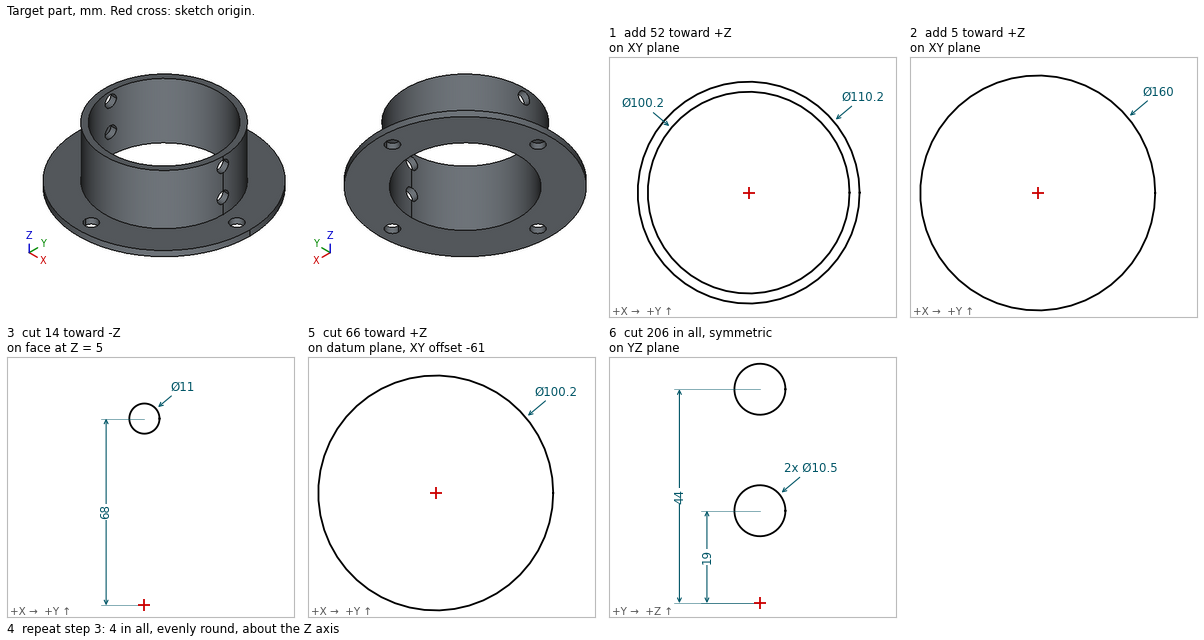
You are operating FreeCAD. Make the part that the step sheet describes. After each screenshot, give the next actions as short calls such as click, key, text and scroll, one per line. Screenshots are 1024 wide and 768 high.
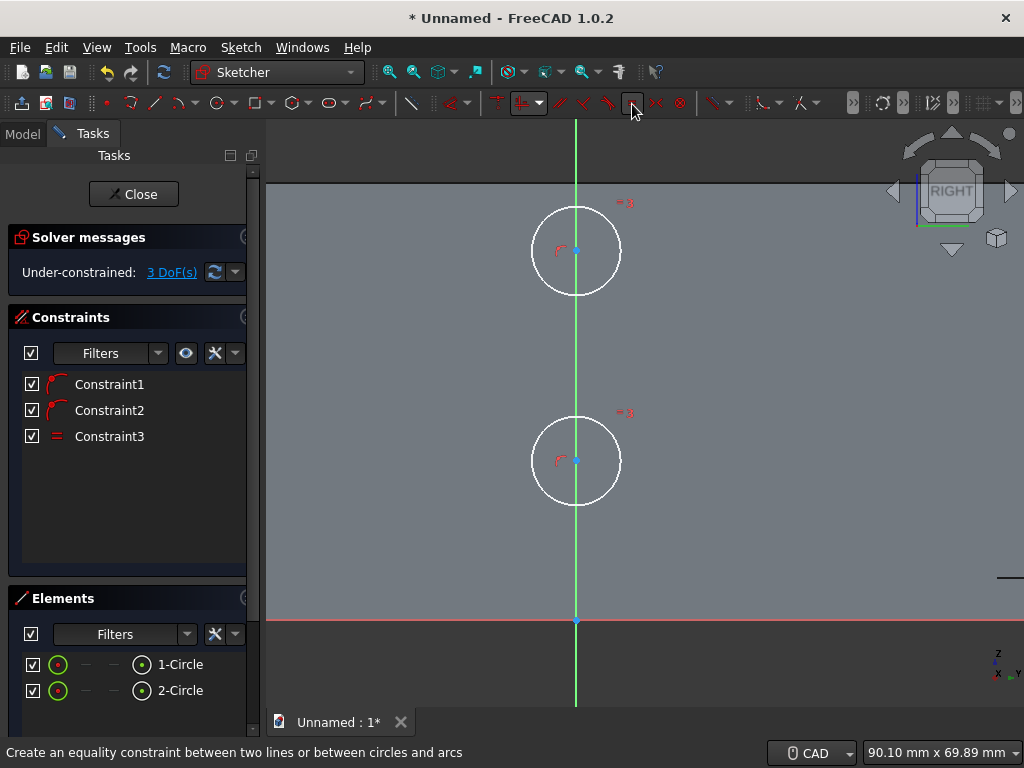
click(450, 104)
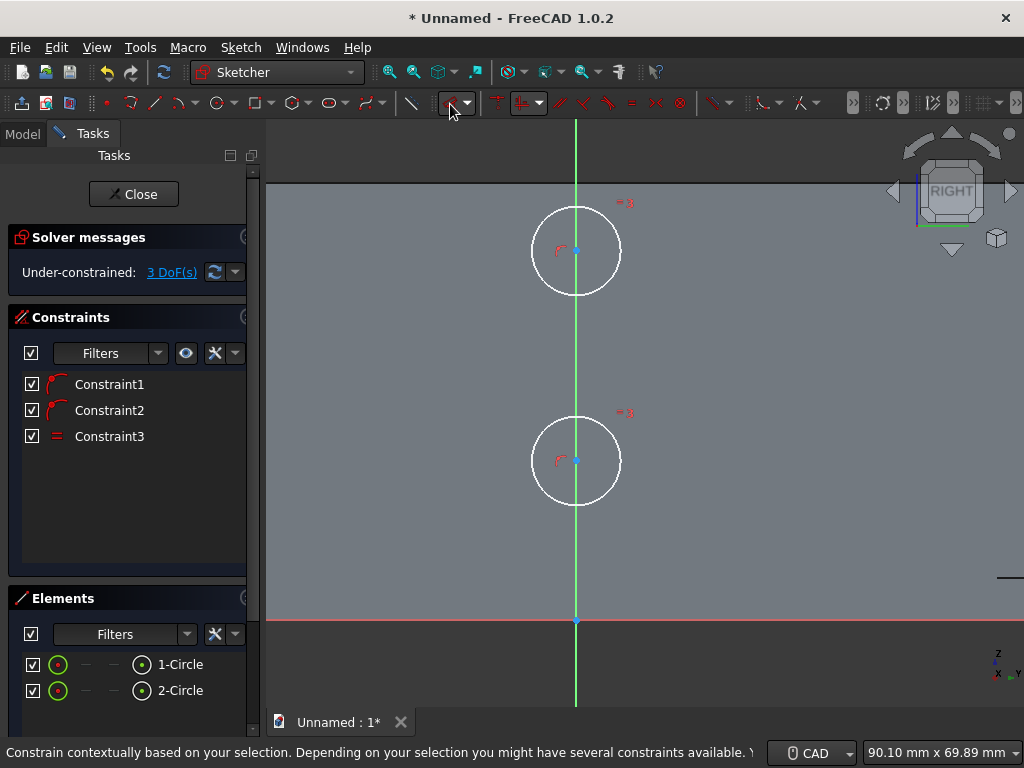
click(608, 430)
click(631, 408)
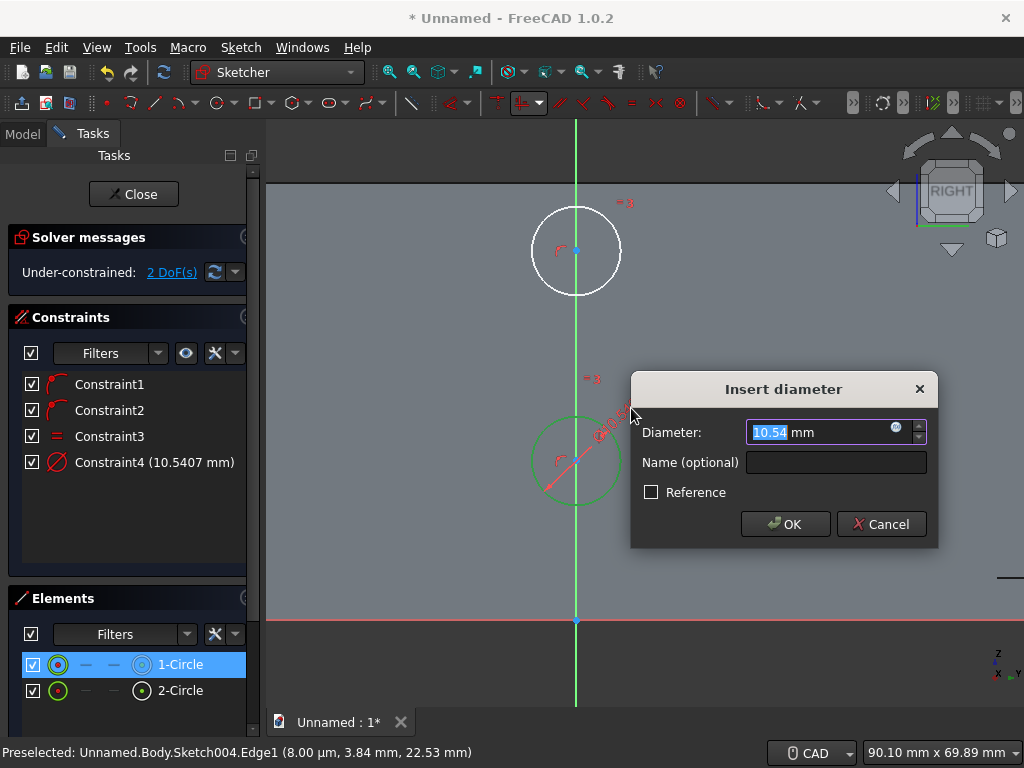
text(10.5)
key(Return)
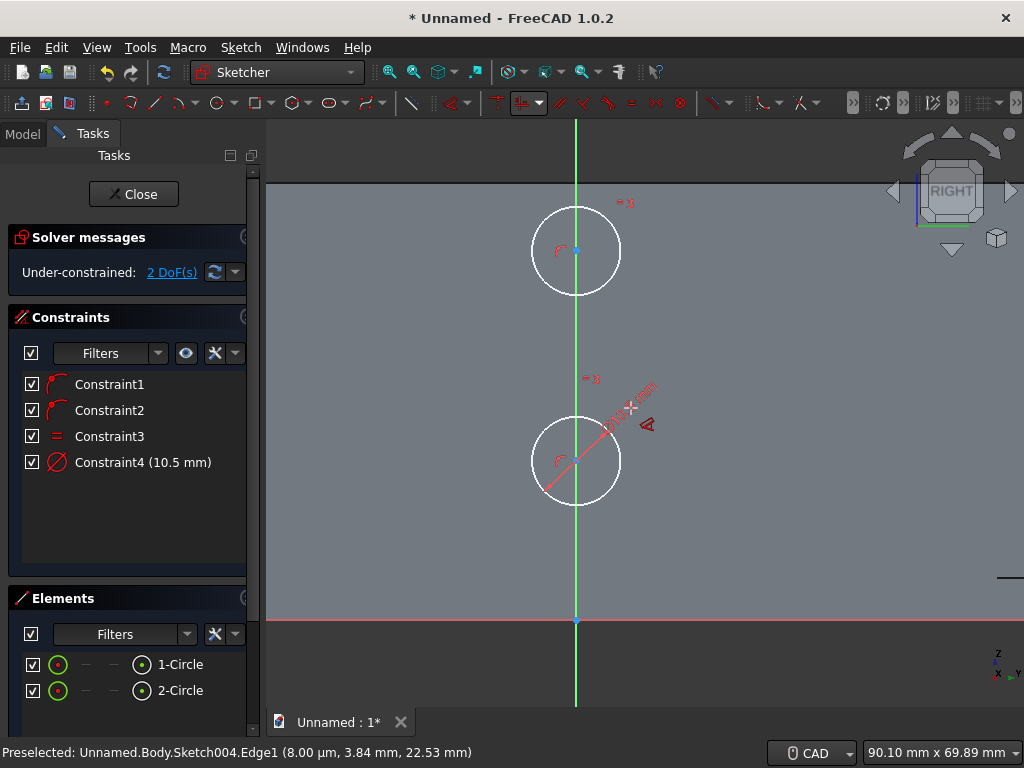
click(576, 461)
click(610, 541)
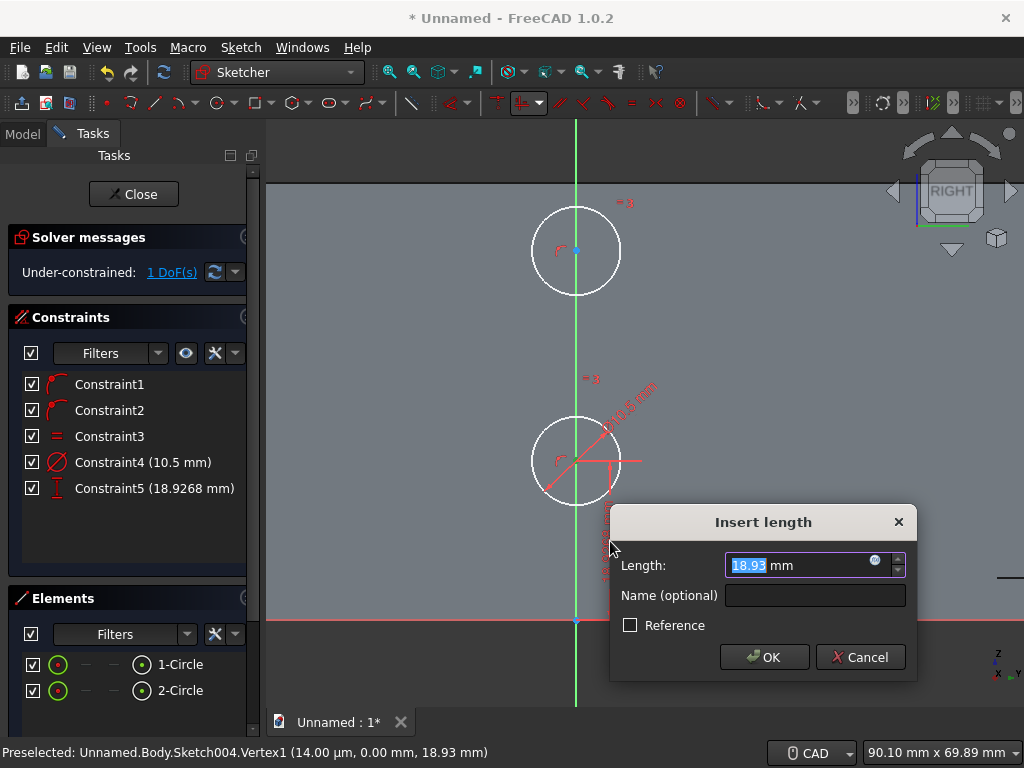
text(19)
key(Return)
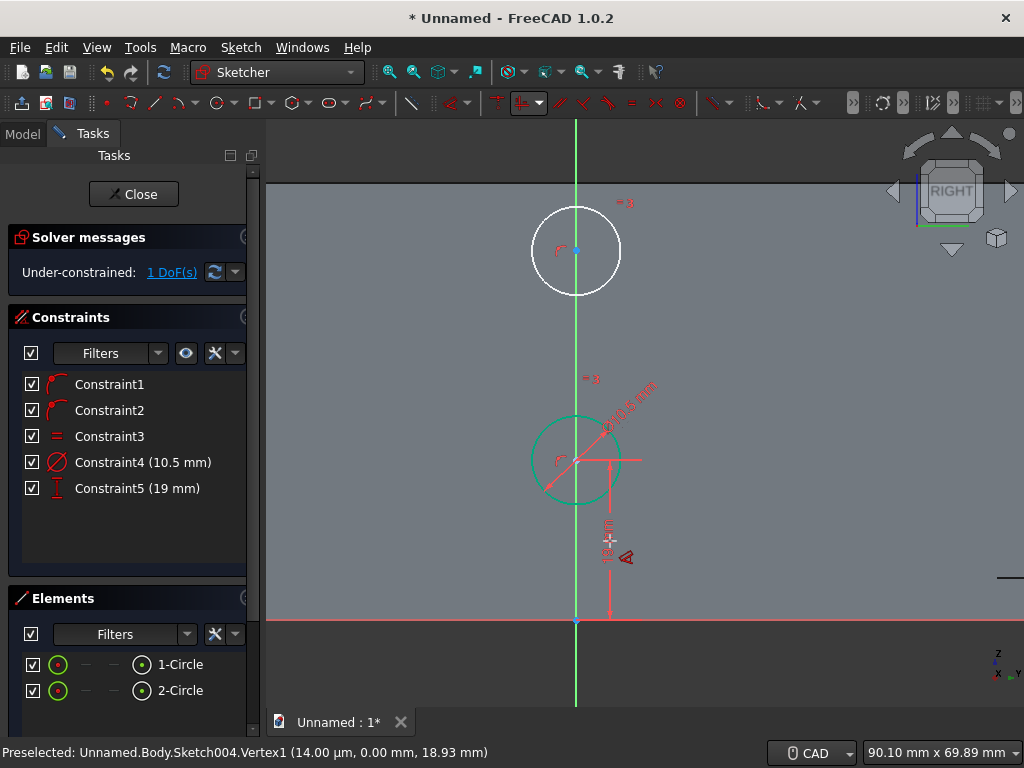
click(576, 251)
click(610, 351)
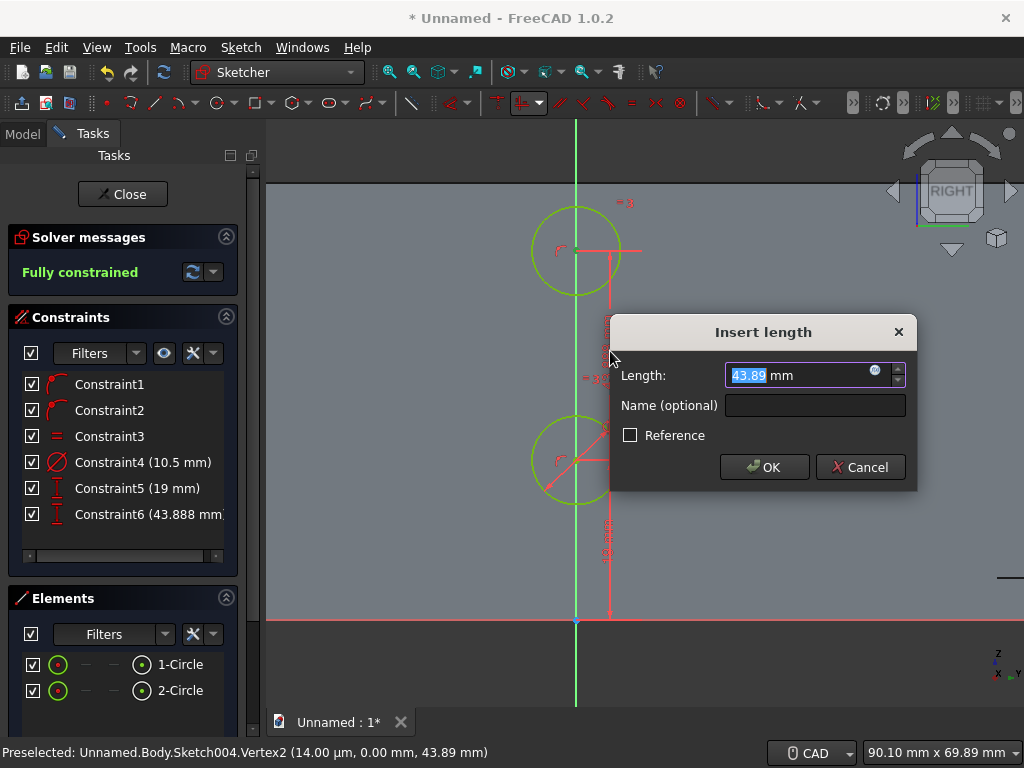
text(44)
key(Return)
key(Escape)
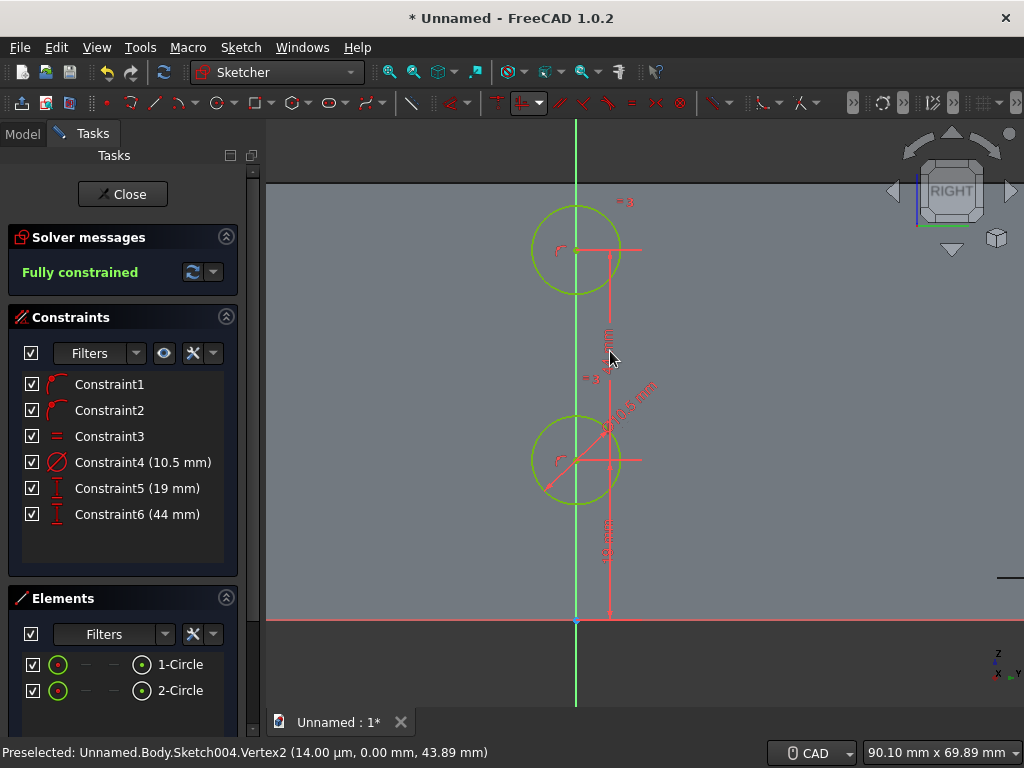
click(123, 194)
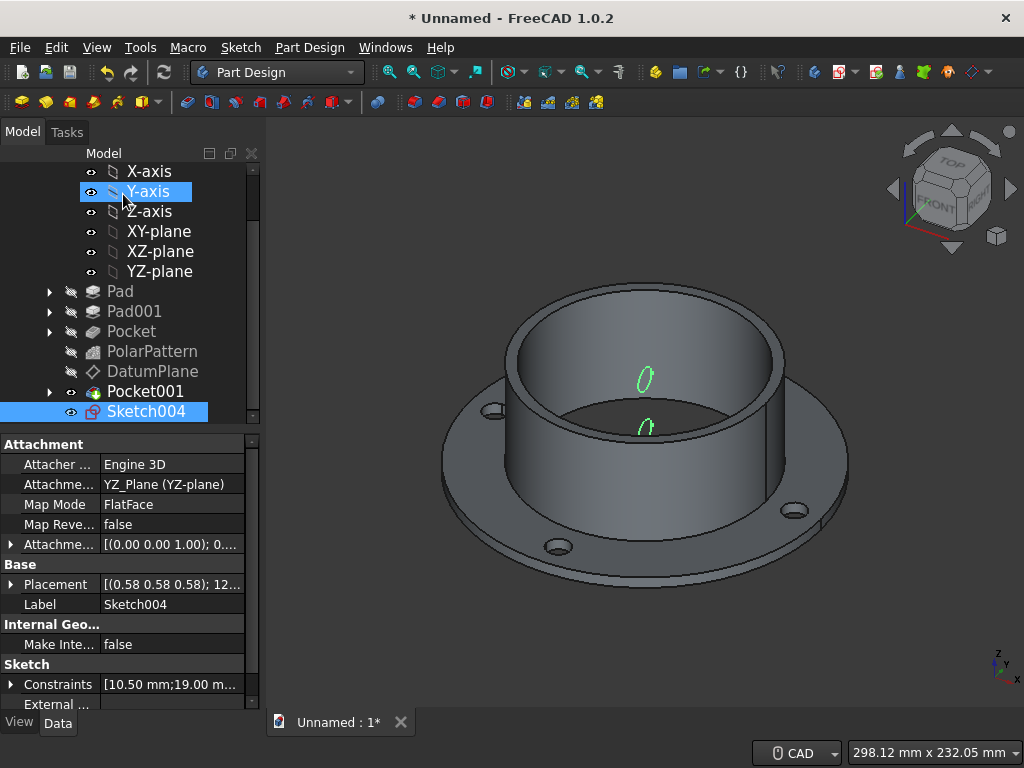
click(188, 102)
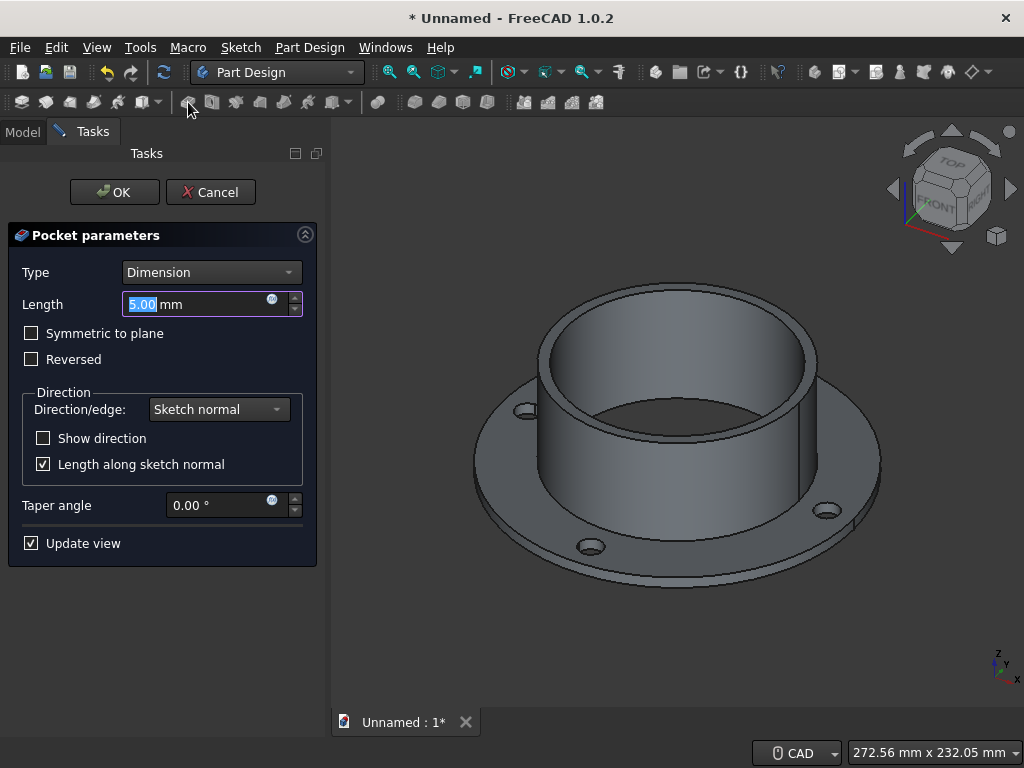
text(206)
key(Tab)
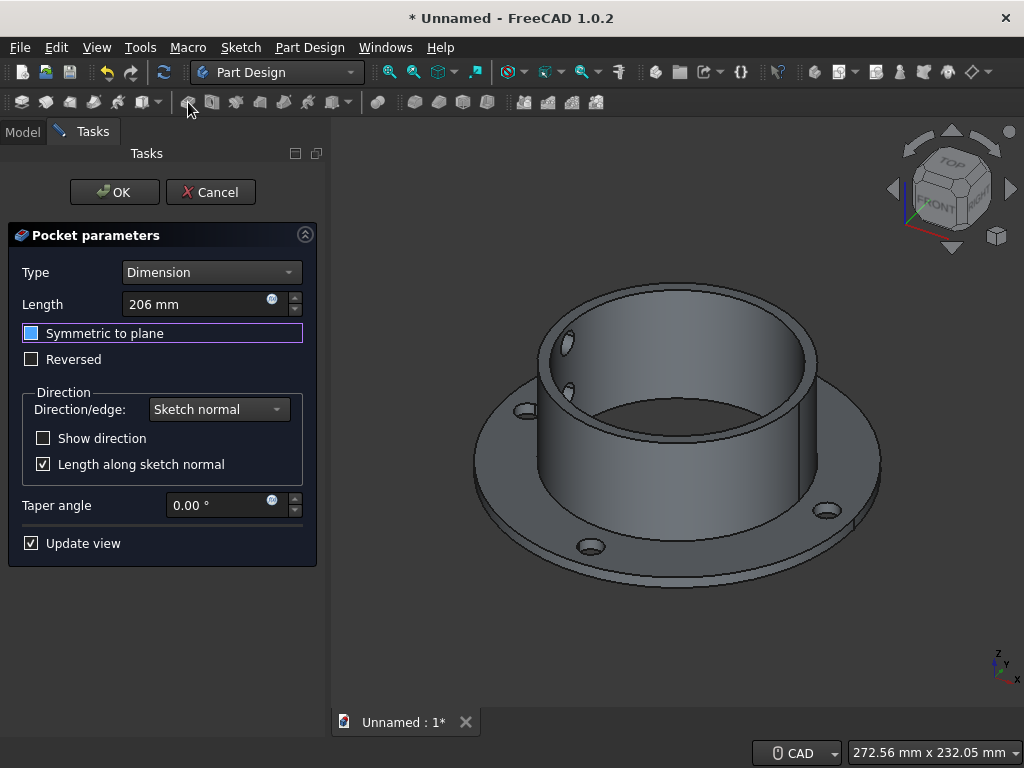
click(30, 333)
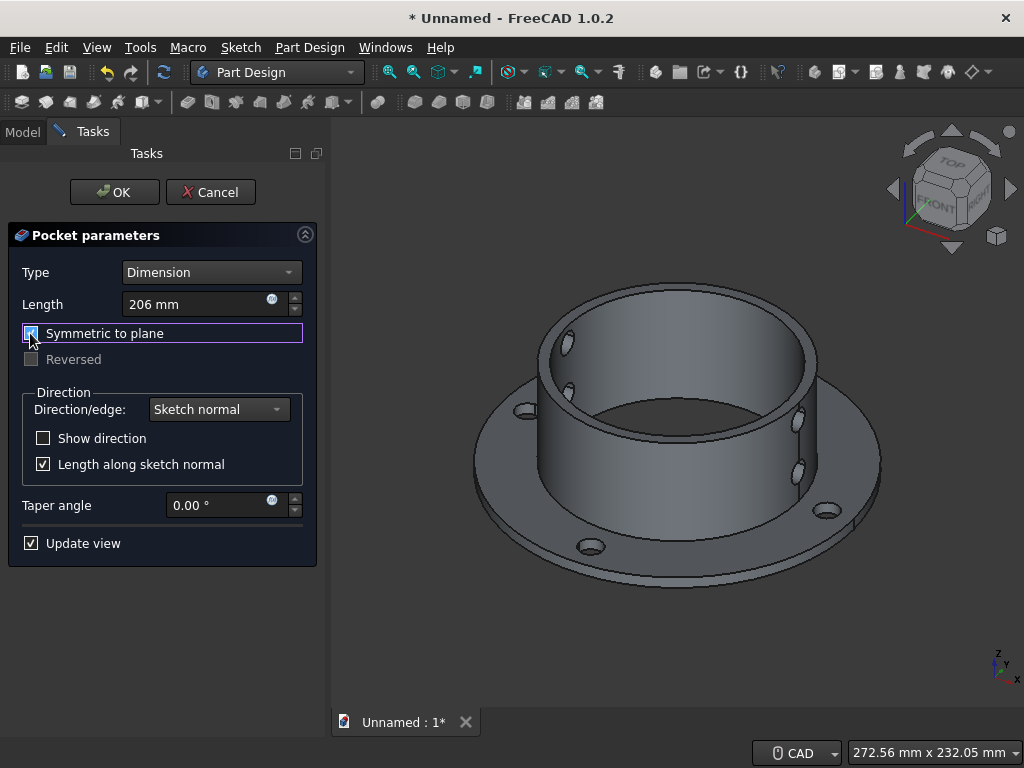
click(115, 192)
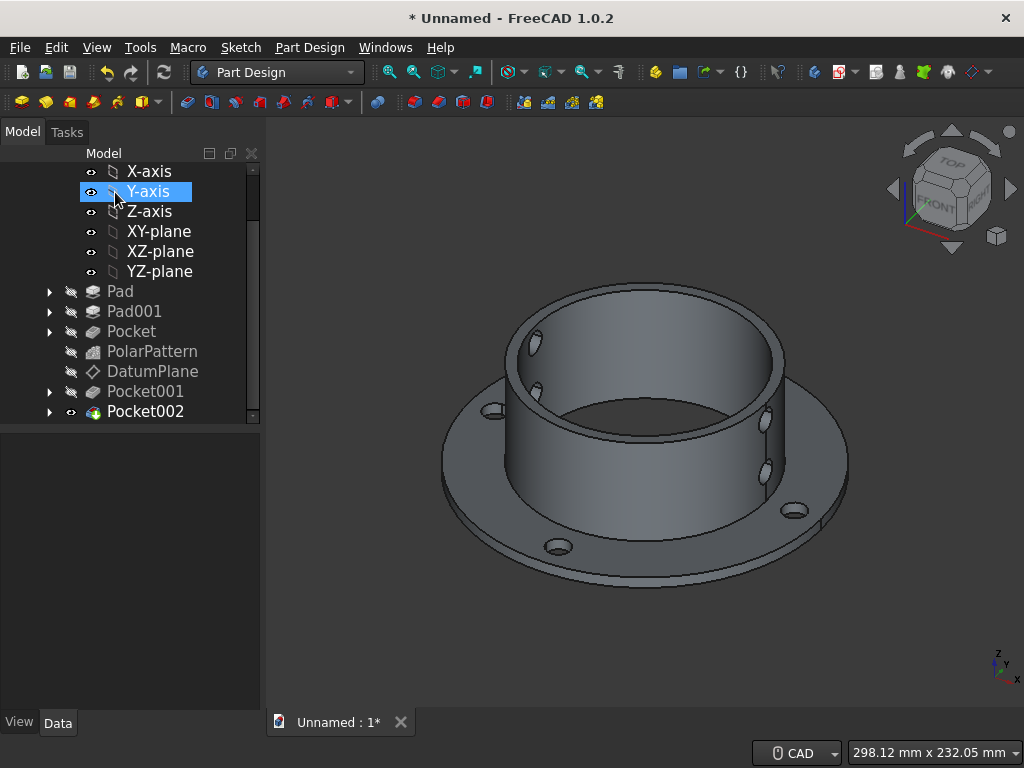
key(0)